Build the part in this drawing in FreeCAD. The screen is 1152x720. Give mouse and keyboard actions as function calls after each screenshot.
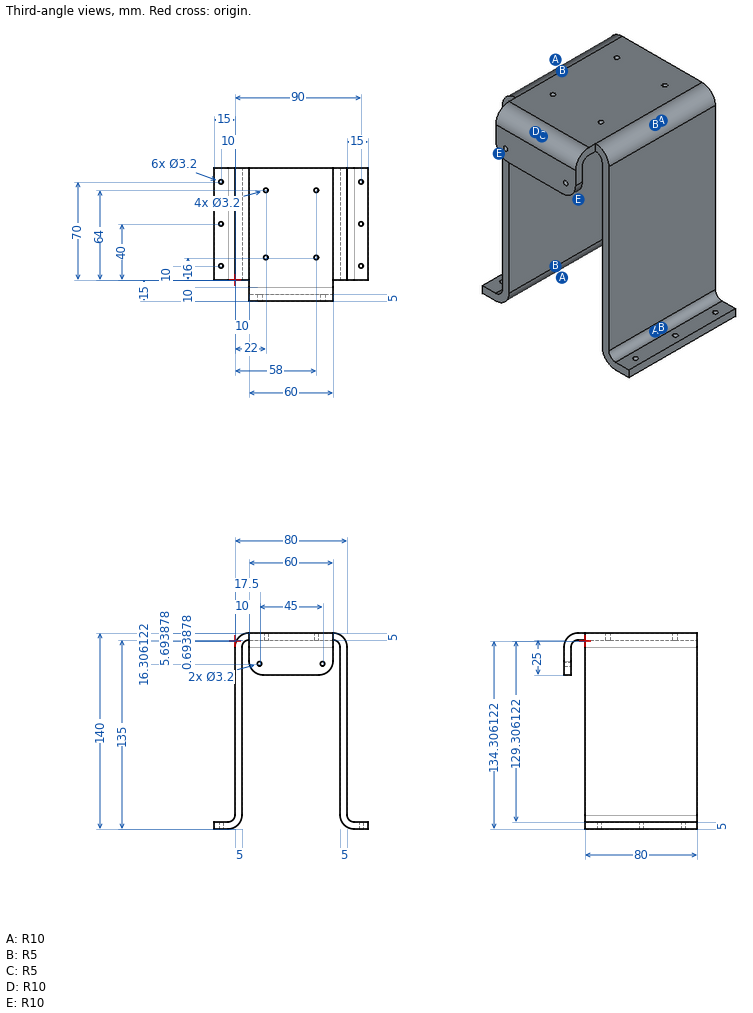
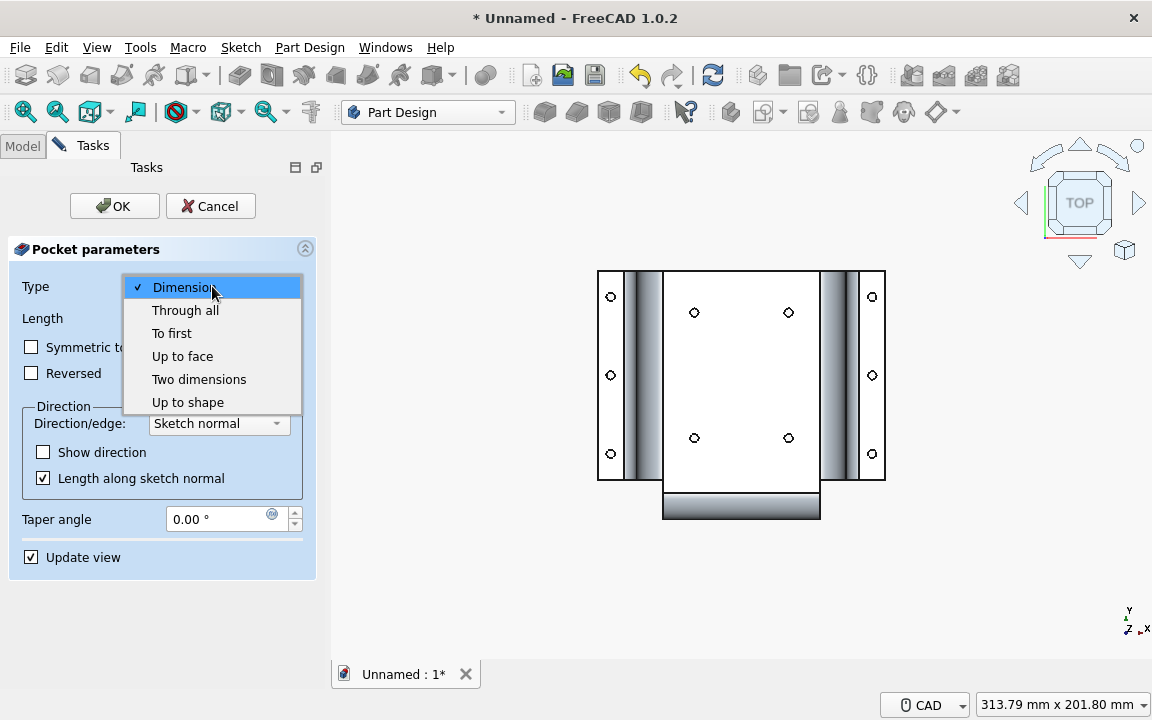
click(212, 310)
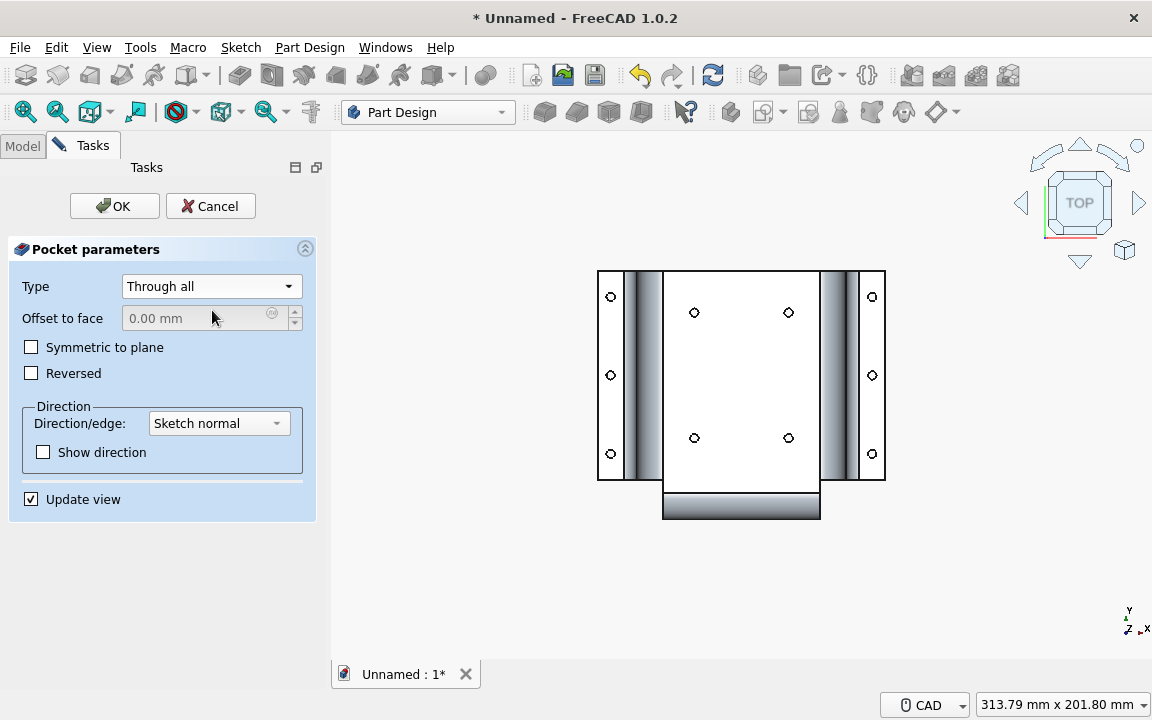
click(115, 206)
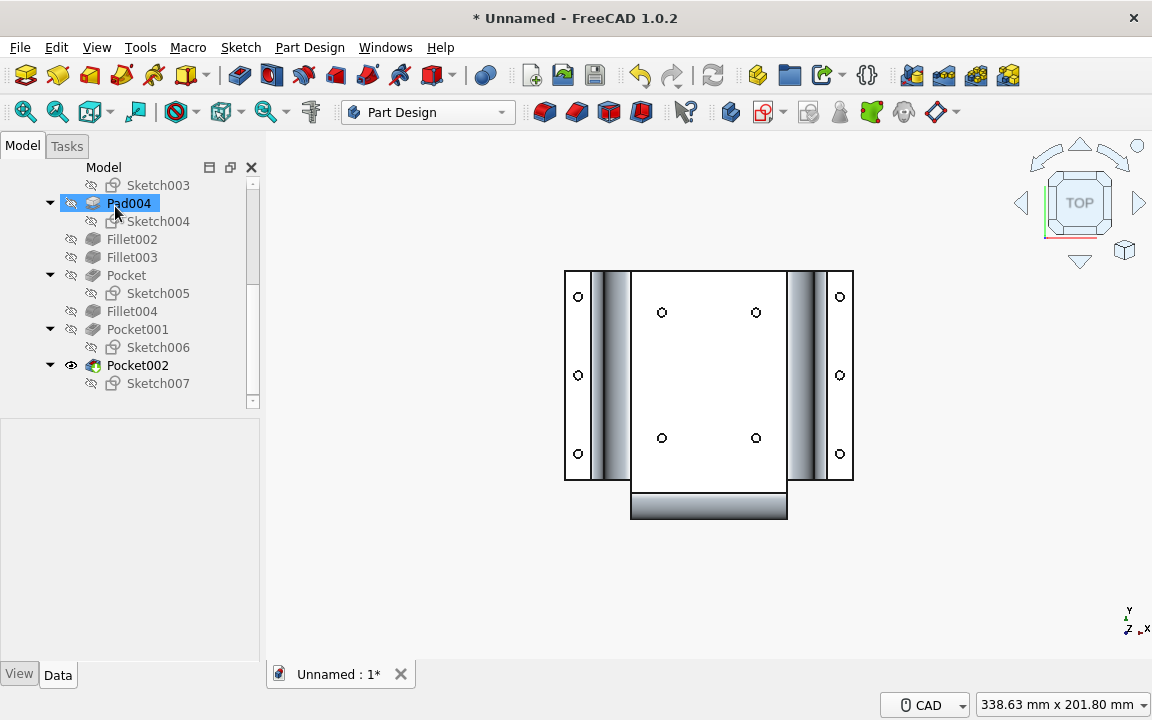
key(0)